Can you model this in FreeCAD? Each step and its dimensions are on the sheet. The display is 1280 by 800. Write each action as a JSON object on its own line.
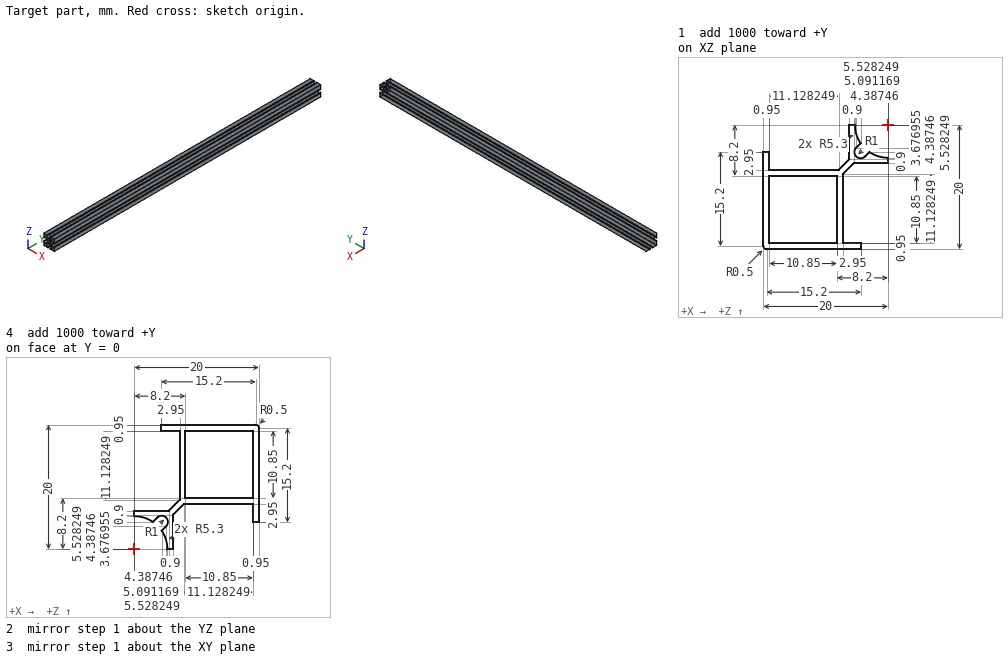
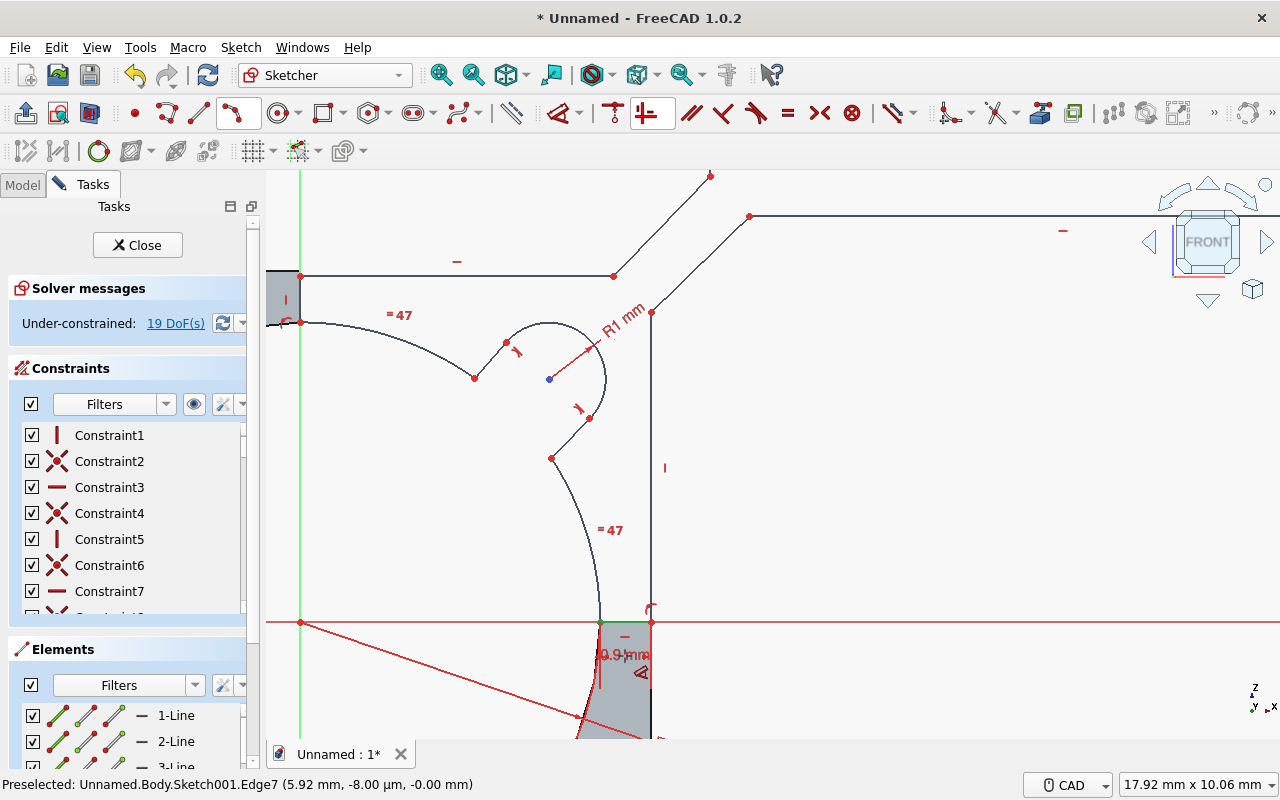
{"action": "left_click", "coordinate": [300, 308]}
{"action": "left_click", "coordinate": [334, 299]}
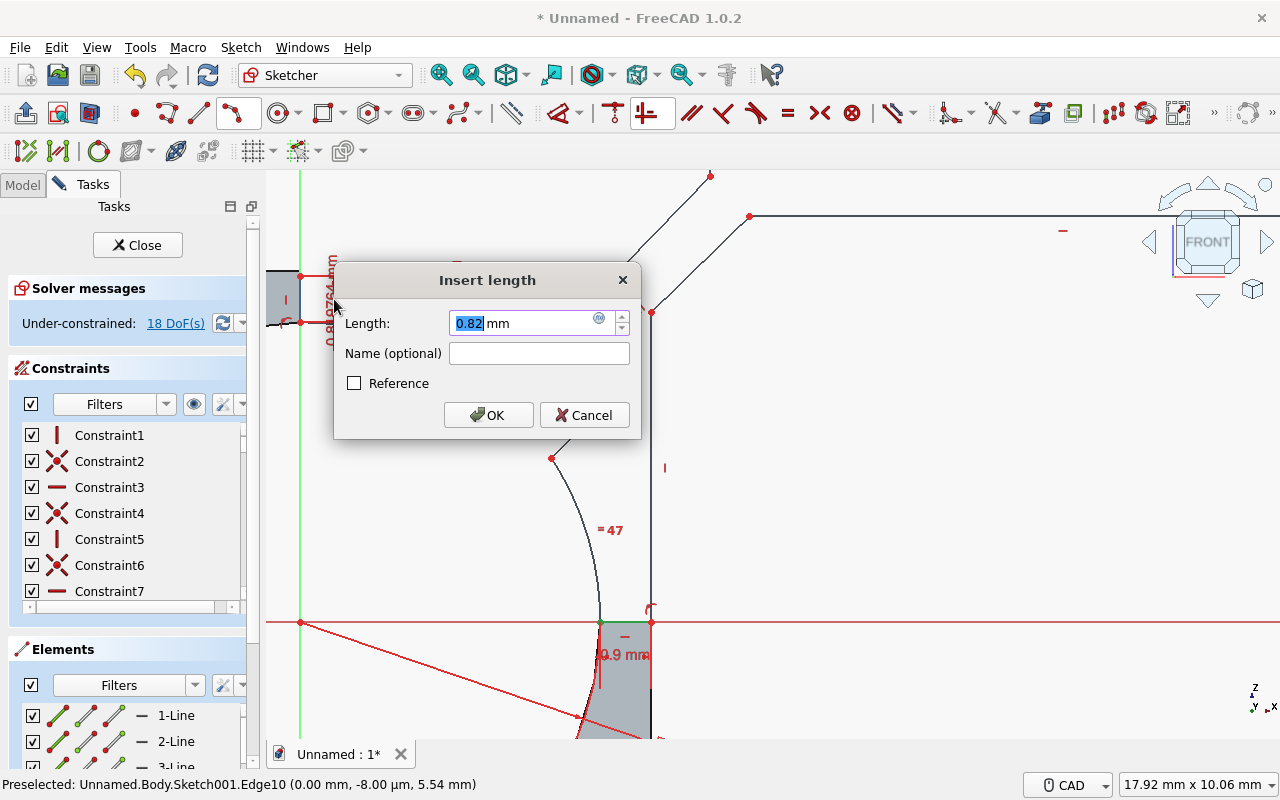
{"action": "type", "text": "0.9"}
{"action": "key", "text": "Return"}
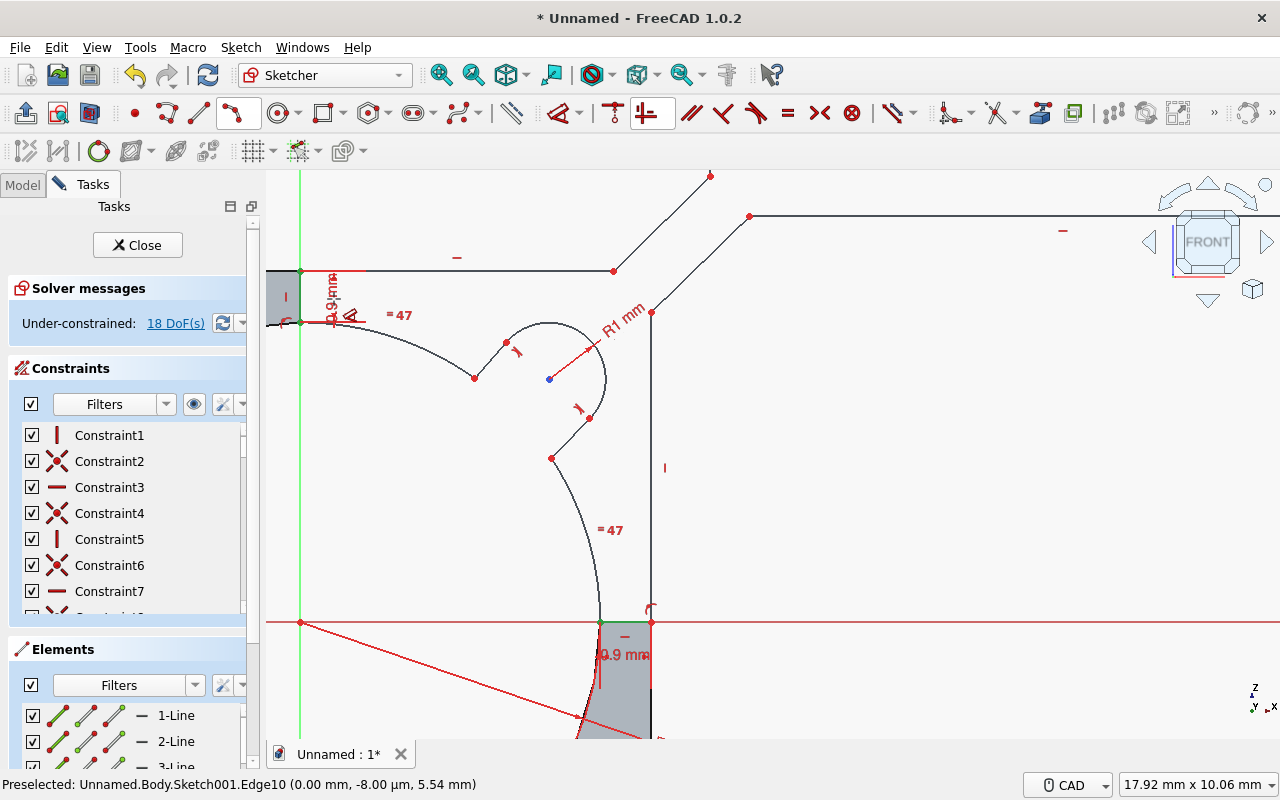
{"action": "scroll", "coordinate": [635, 626], "scroll_direction": "down", "scroll_amount": 6}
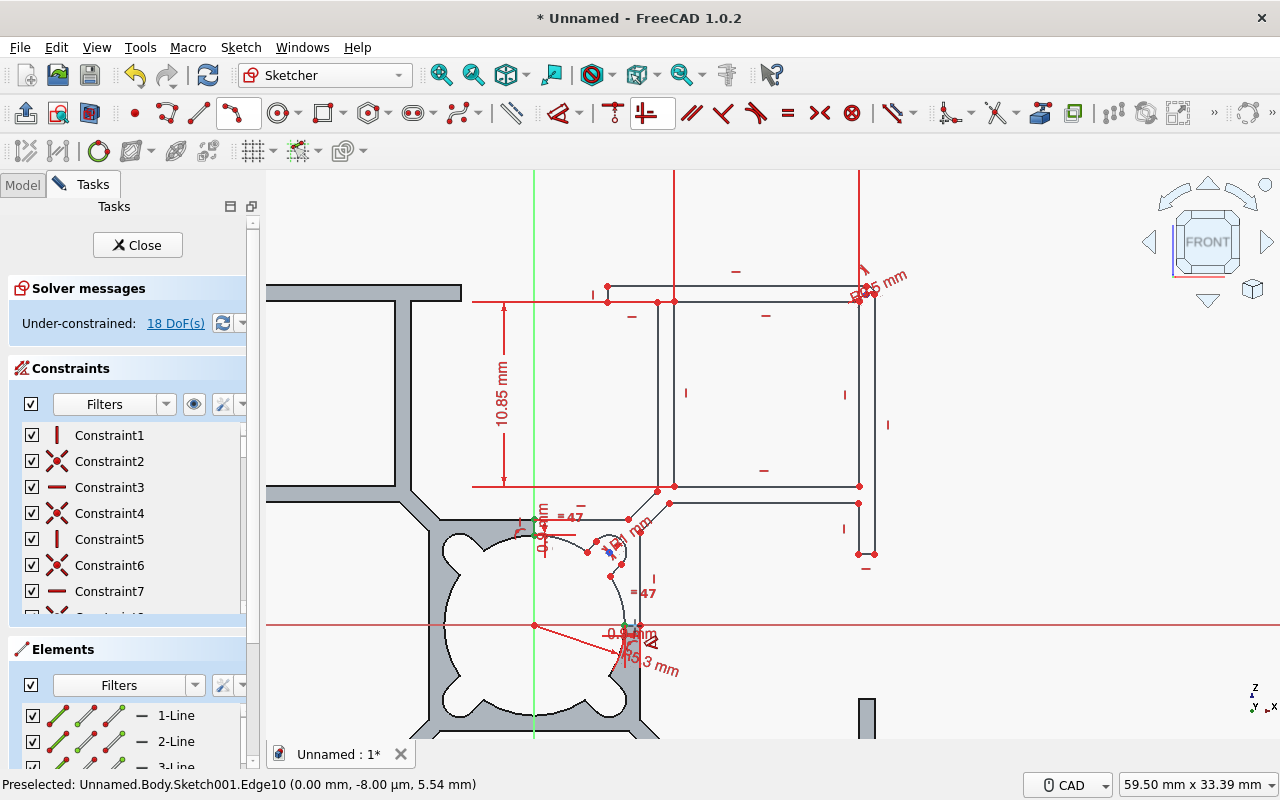
{"action": "scroll", "coordinate": [875, 295], "scroll_direction": "up", "scroll_amount": 2}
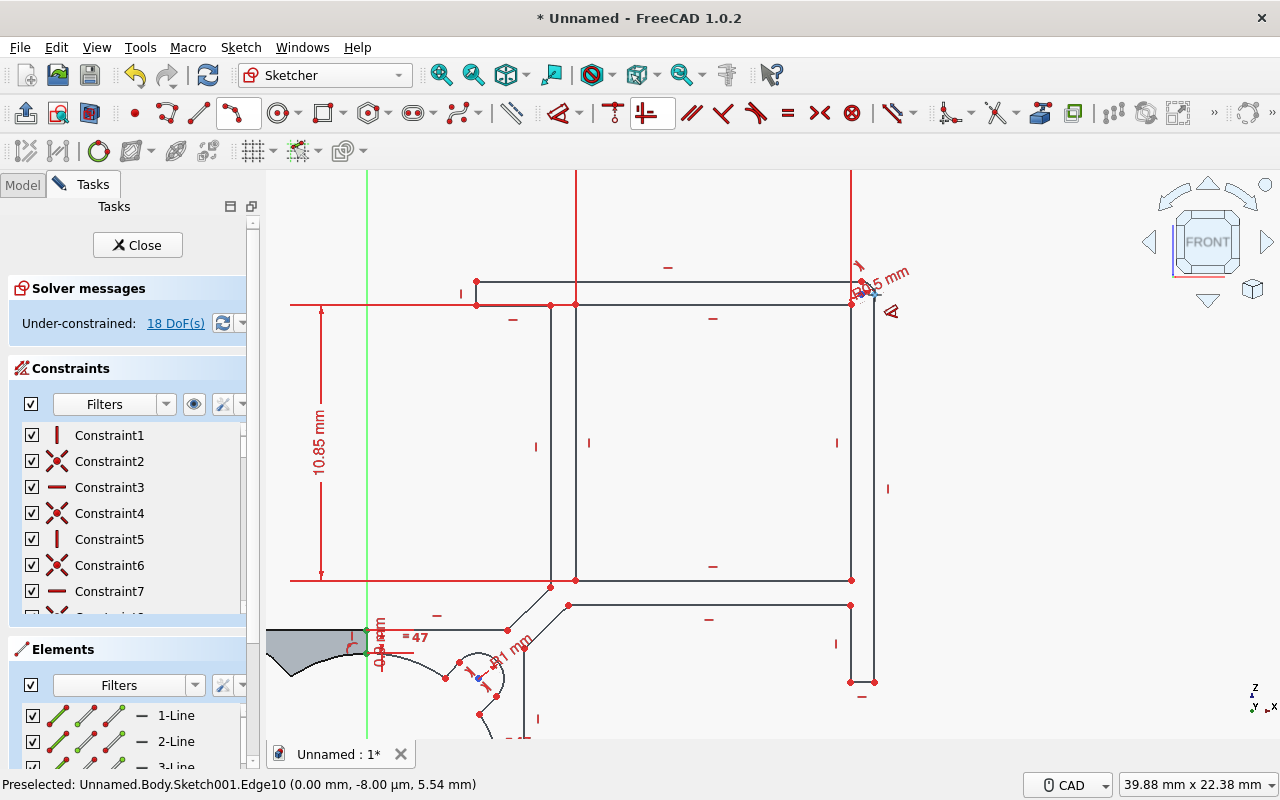
{"action": "left_click", "coordinate": [874, 294]}
{"action": "left_click", "coordinate": [620, 260]}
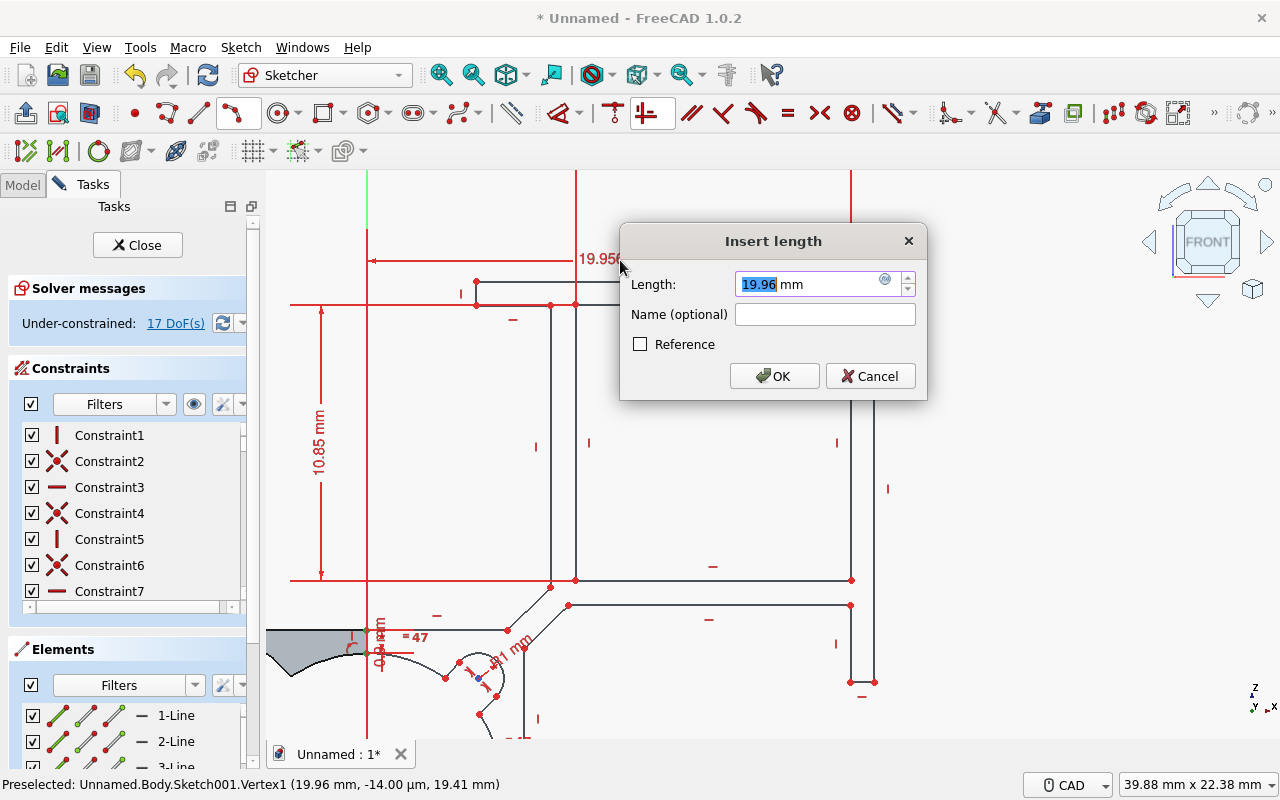
{"action": "type", "text": "20"}
{"action": "key", "text": "Return"}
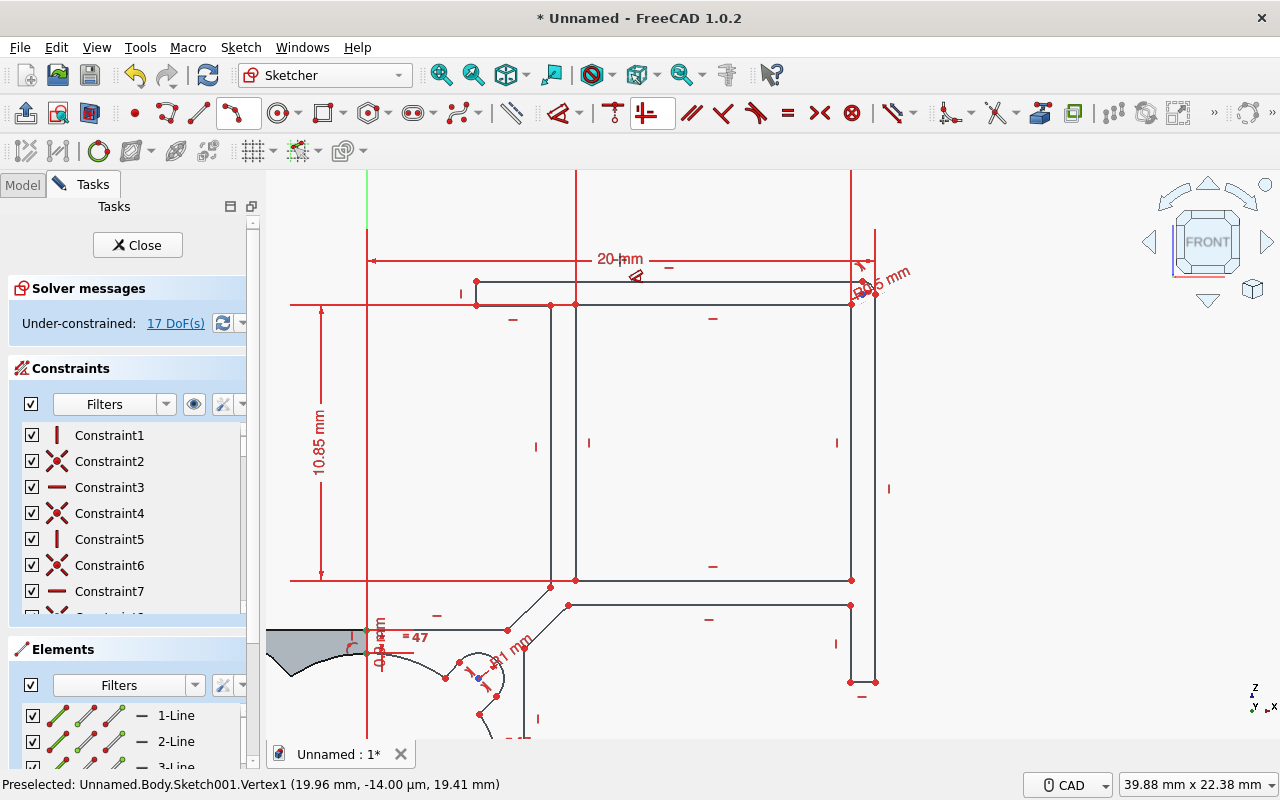
{"action": "left_click", "coordinate": [476, 282]}
{"action": "left_click", "coordinate": [333, 496]}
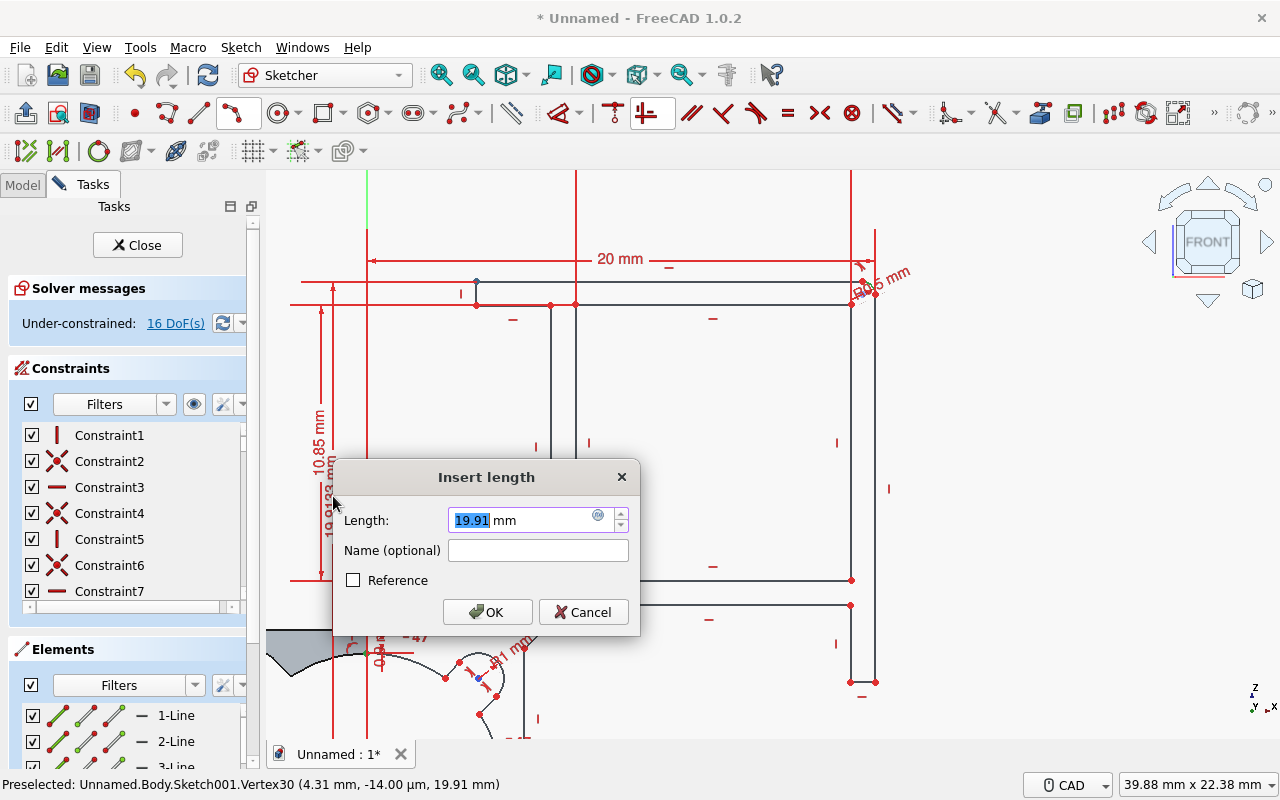
{"action": "type", "text": "20"}
{"action": "key", "text": "Return"}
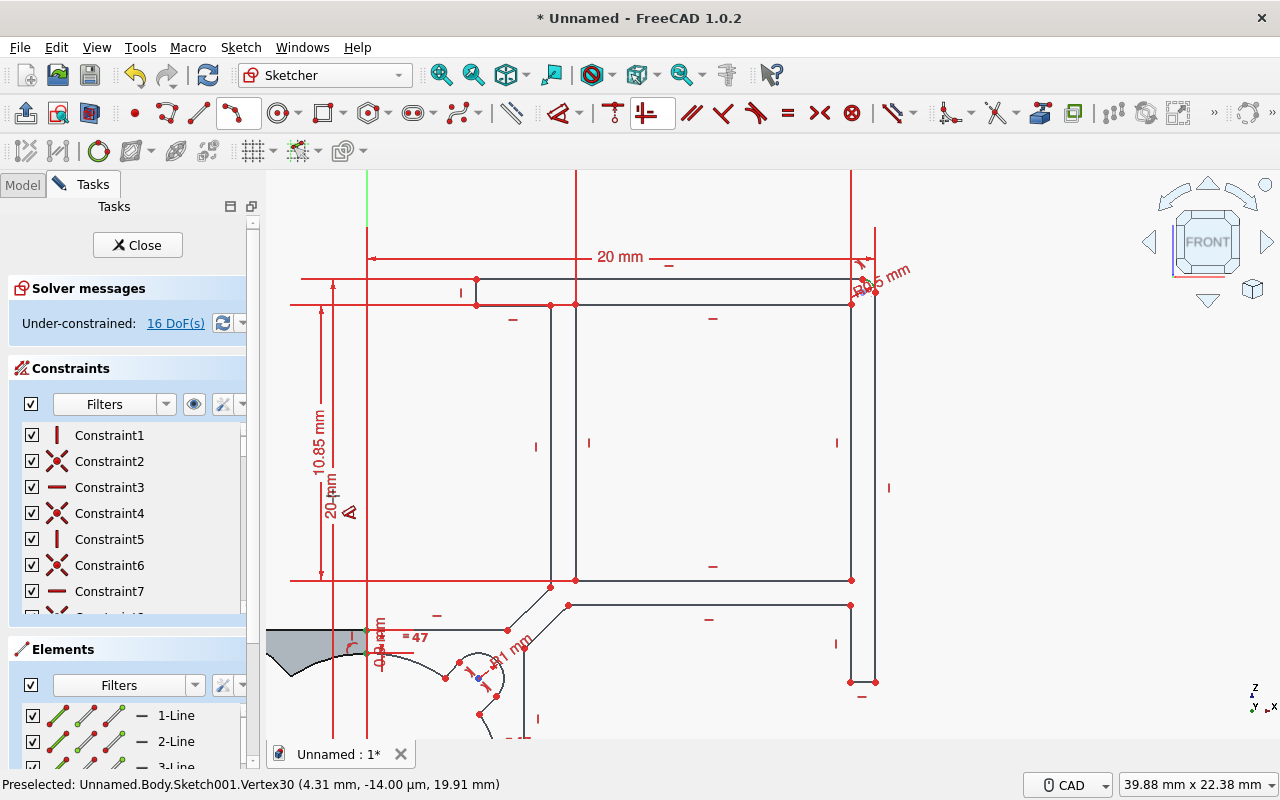
{"action": "left_click", "coordinate": [875, 409]}
{"action": "left_click", "coordinate": [909, 487]}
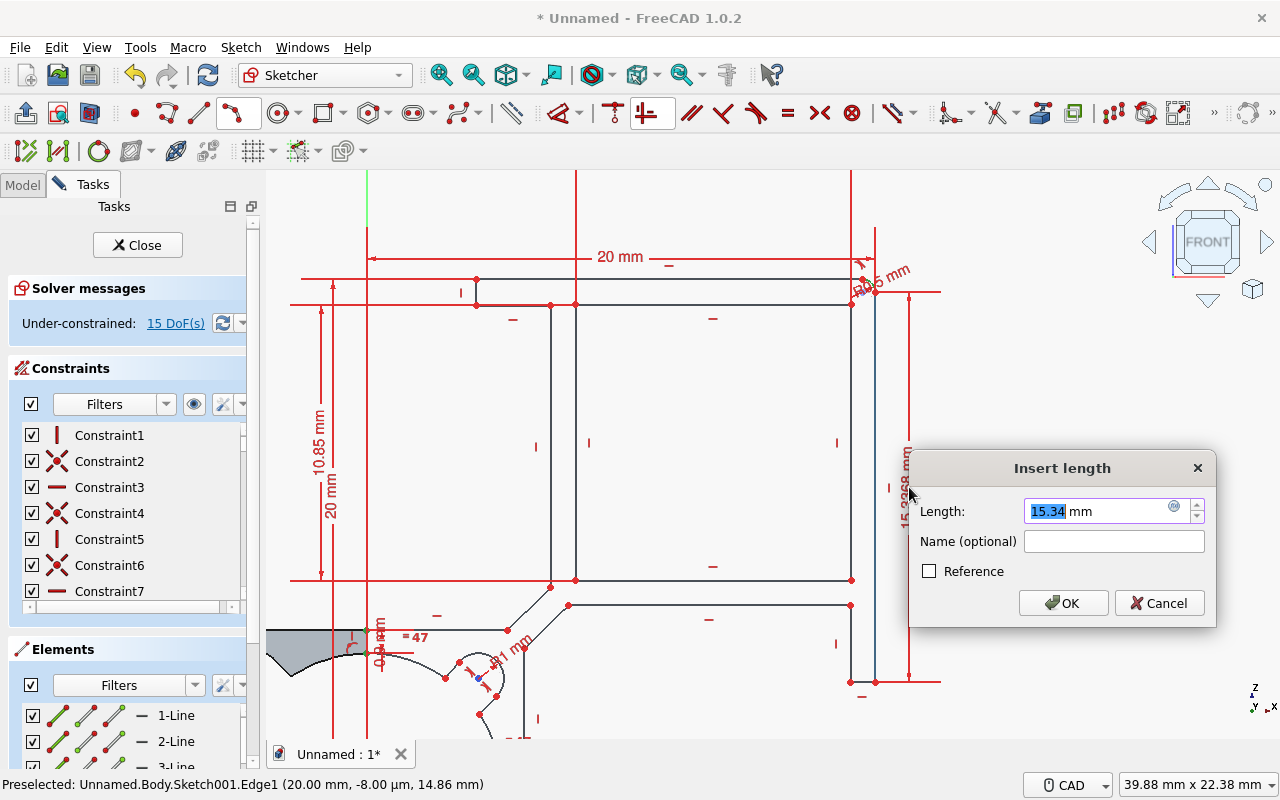
{"action": "type", "text": "15.2"}
{"action": "key", "text": "Return"}